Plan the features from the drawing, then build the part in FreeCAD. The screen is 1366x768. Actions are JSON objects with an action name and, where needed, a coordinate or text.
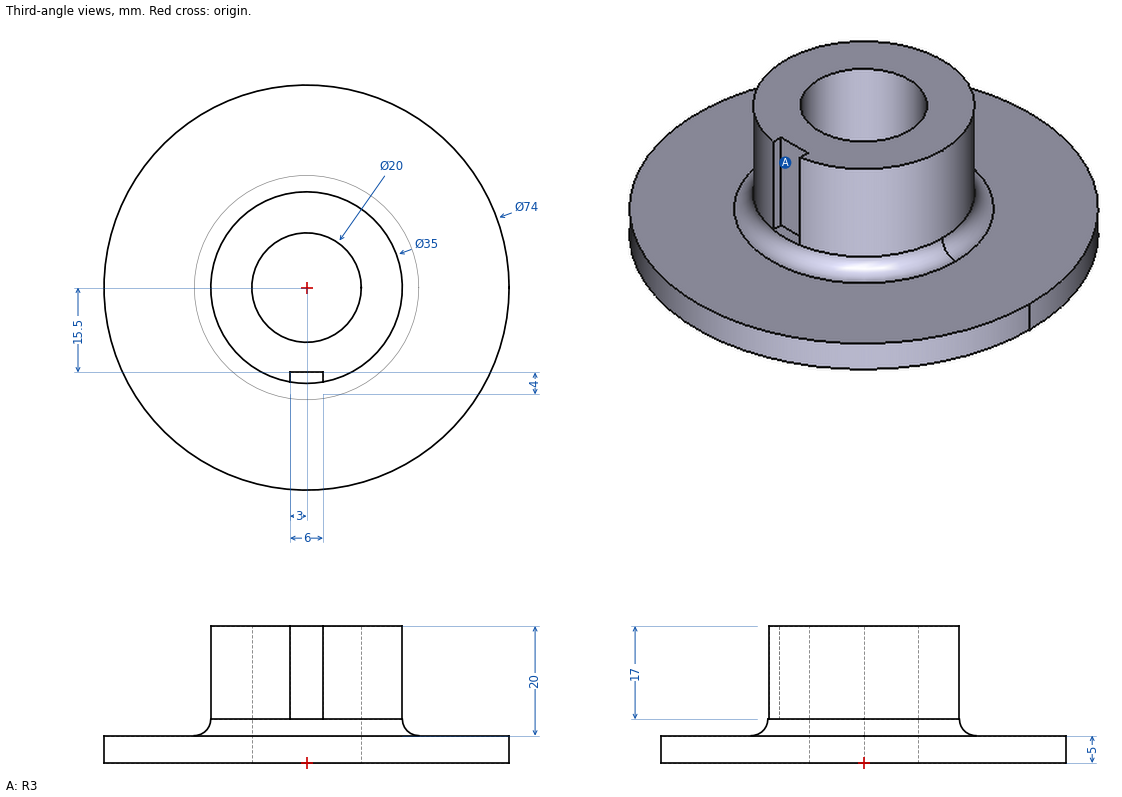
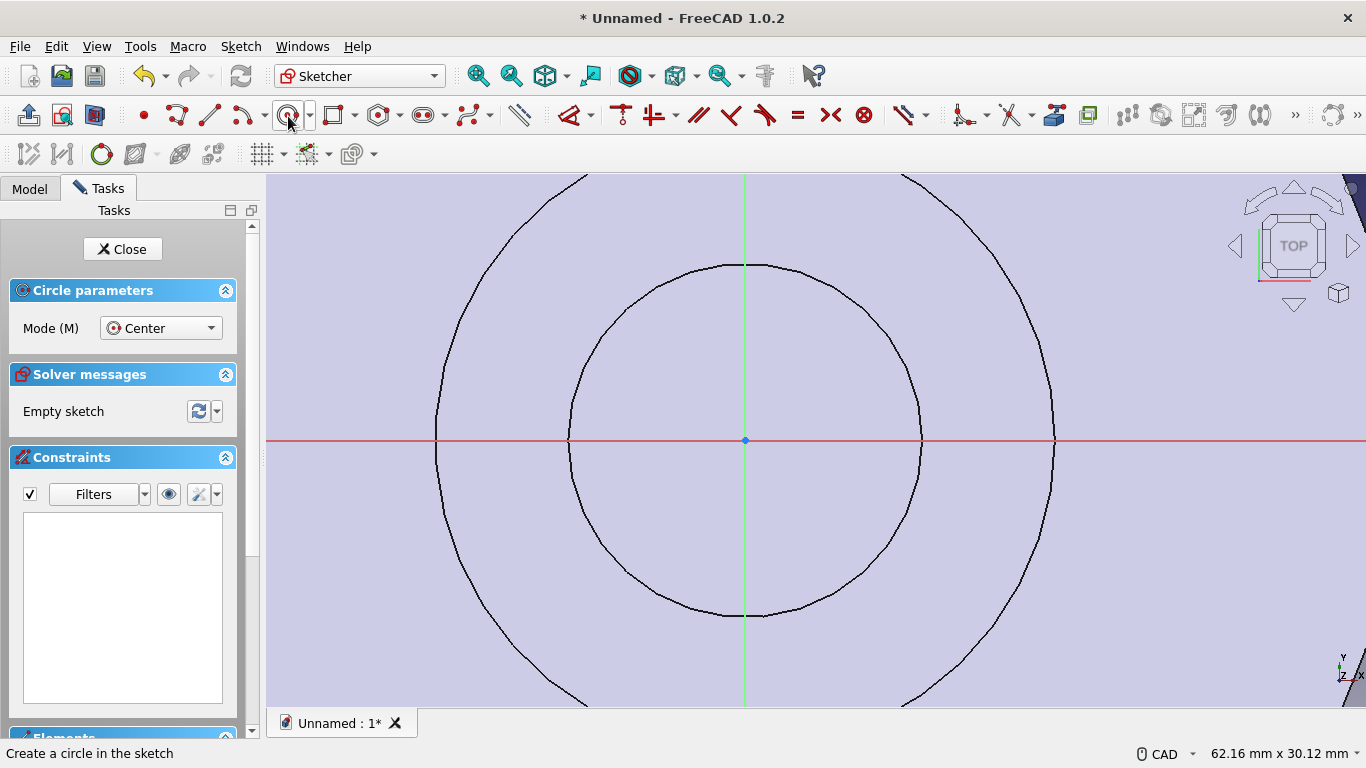
{"action": "left_click", "coordinate": [745, 440]}
{"action": "mouse_move", "coordinate": [870, 315]}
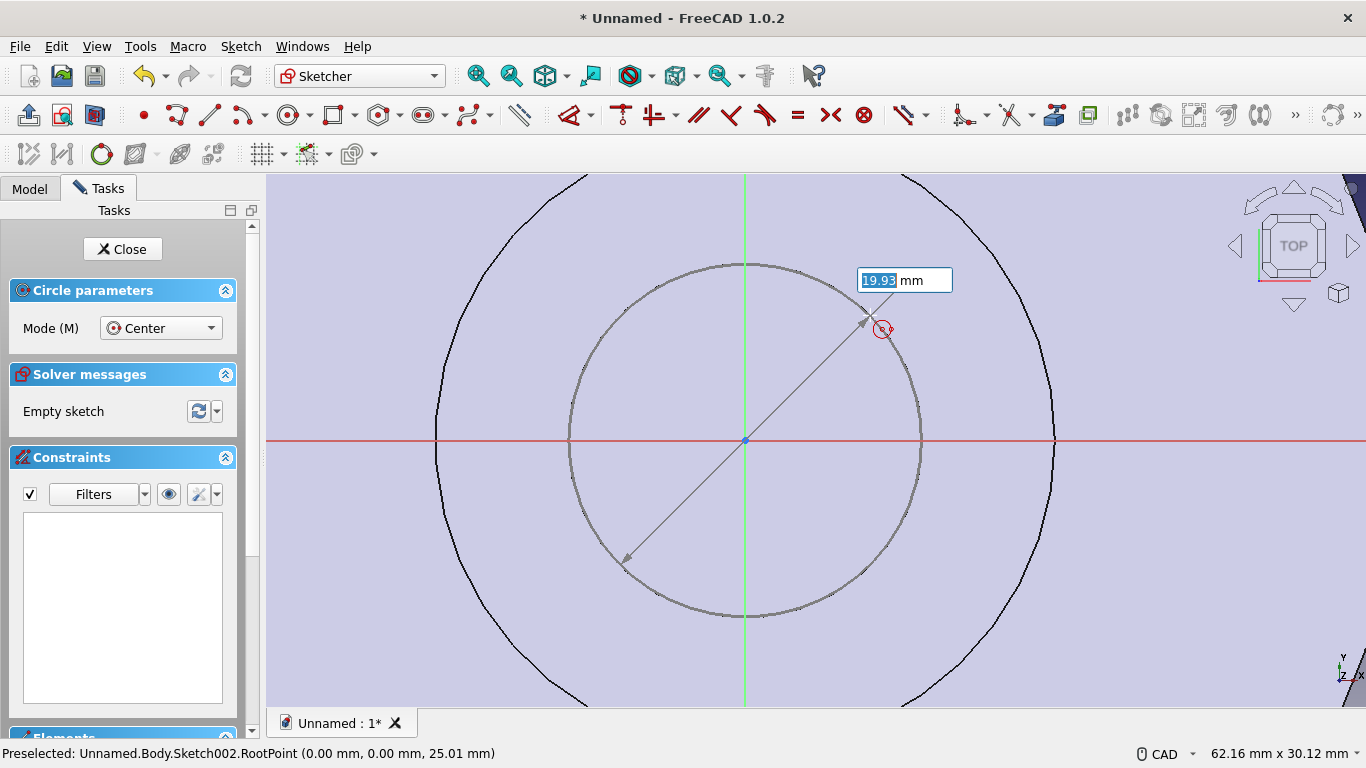
{"action": "type", "text": "20"}
{"action": "key", "text": "Return"}
{"action": "key", "text": "Escape"}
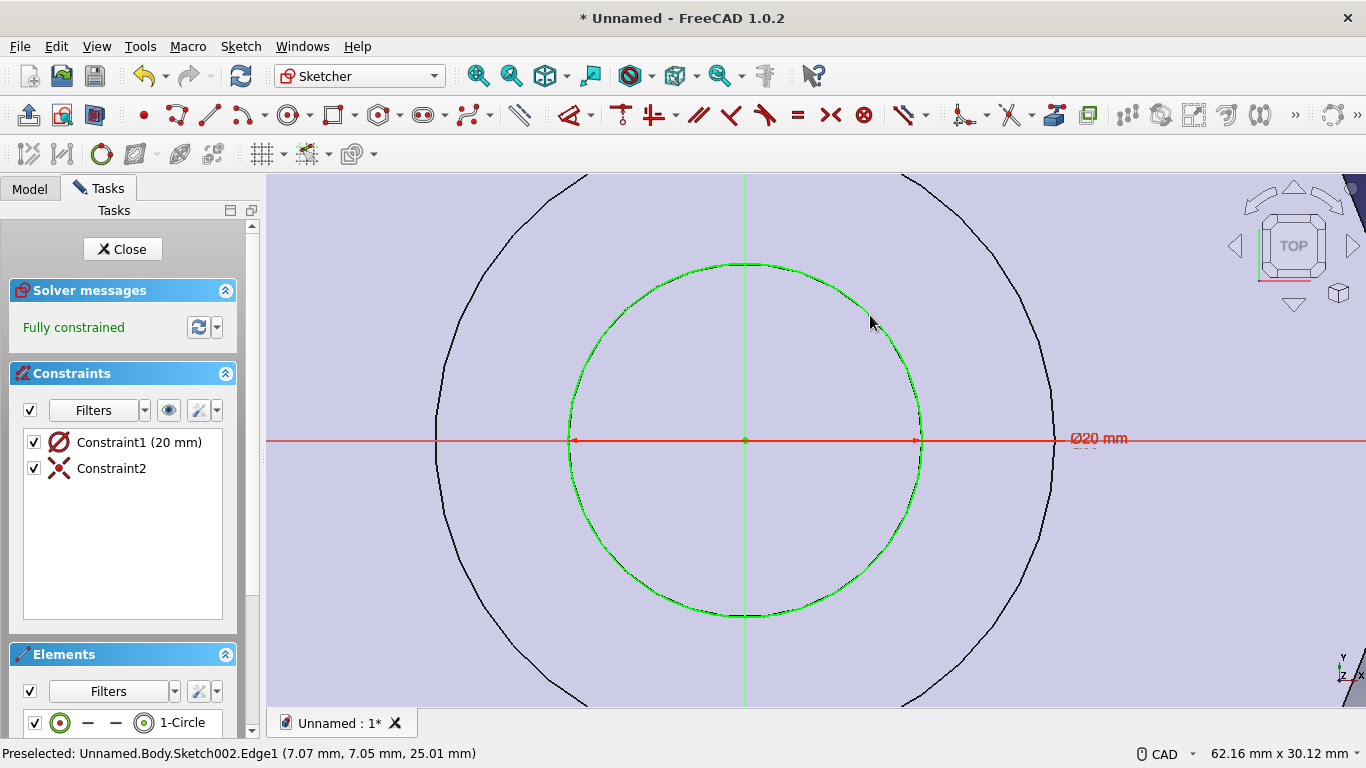
{"action": "left_click", "coordinate": [123, 249]}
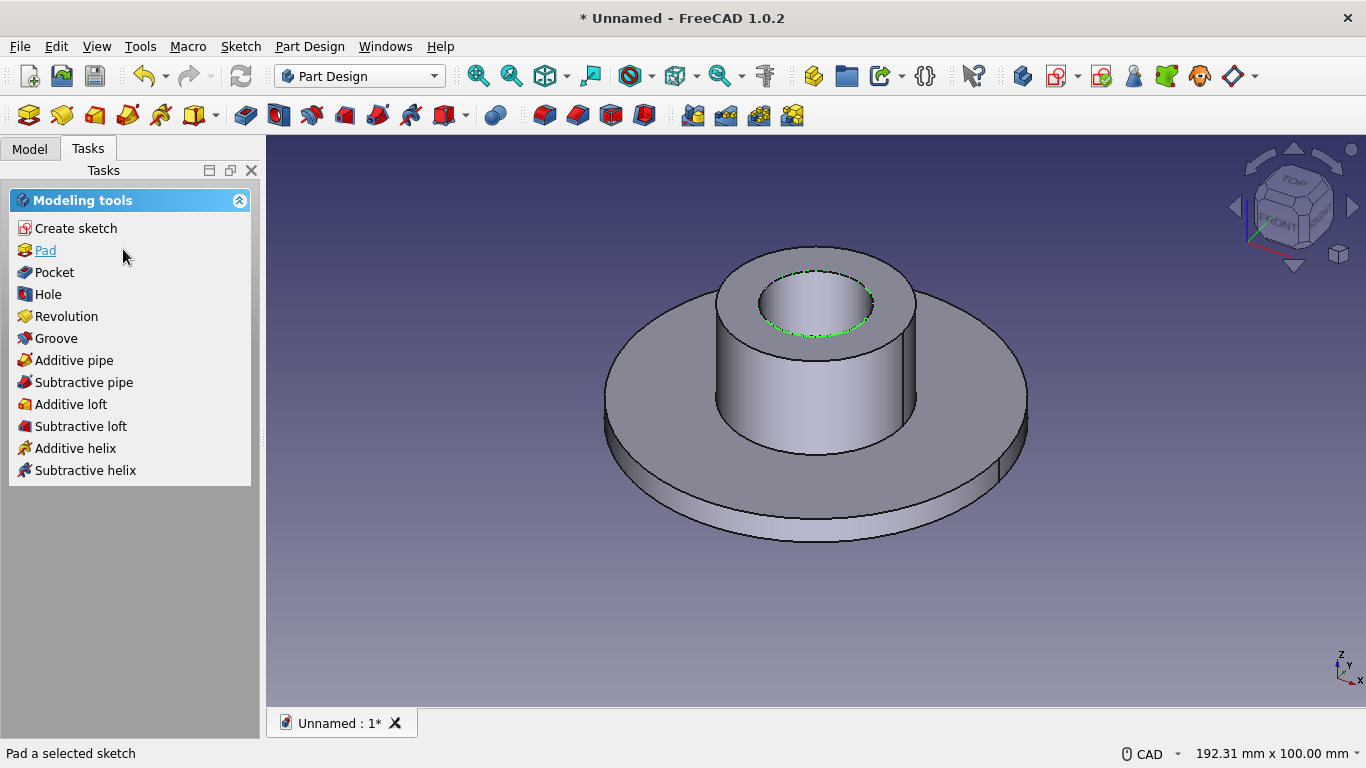
{"action": "left_click", "coordinate": [246, 116]}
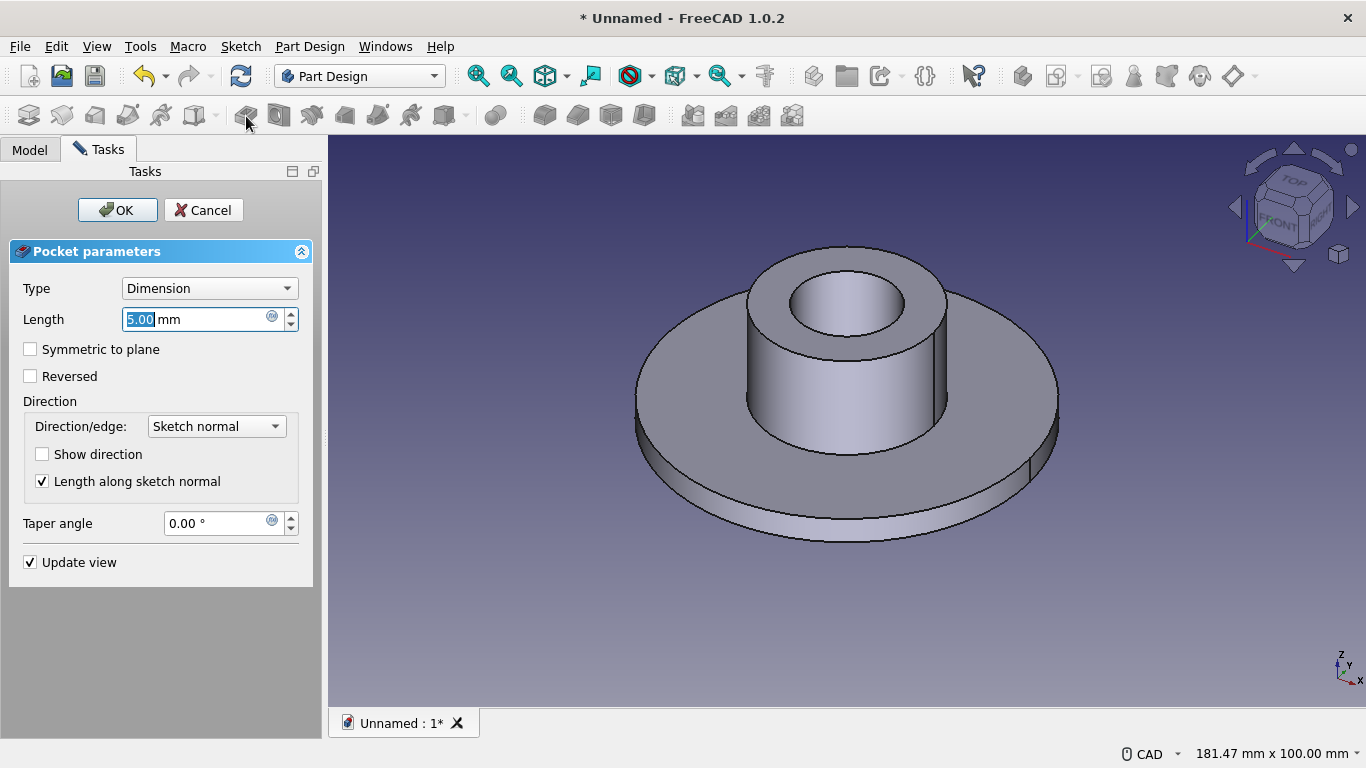
{"action": "left_click", "coordinate": [210, 288]}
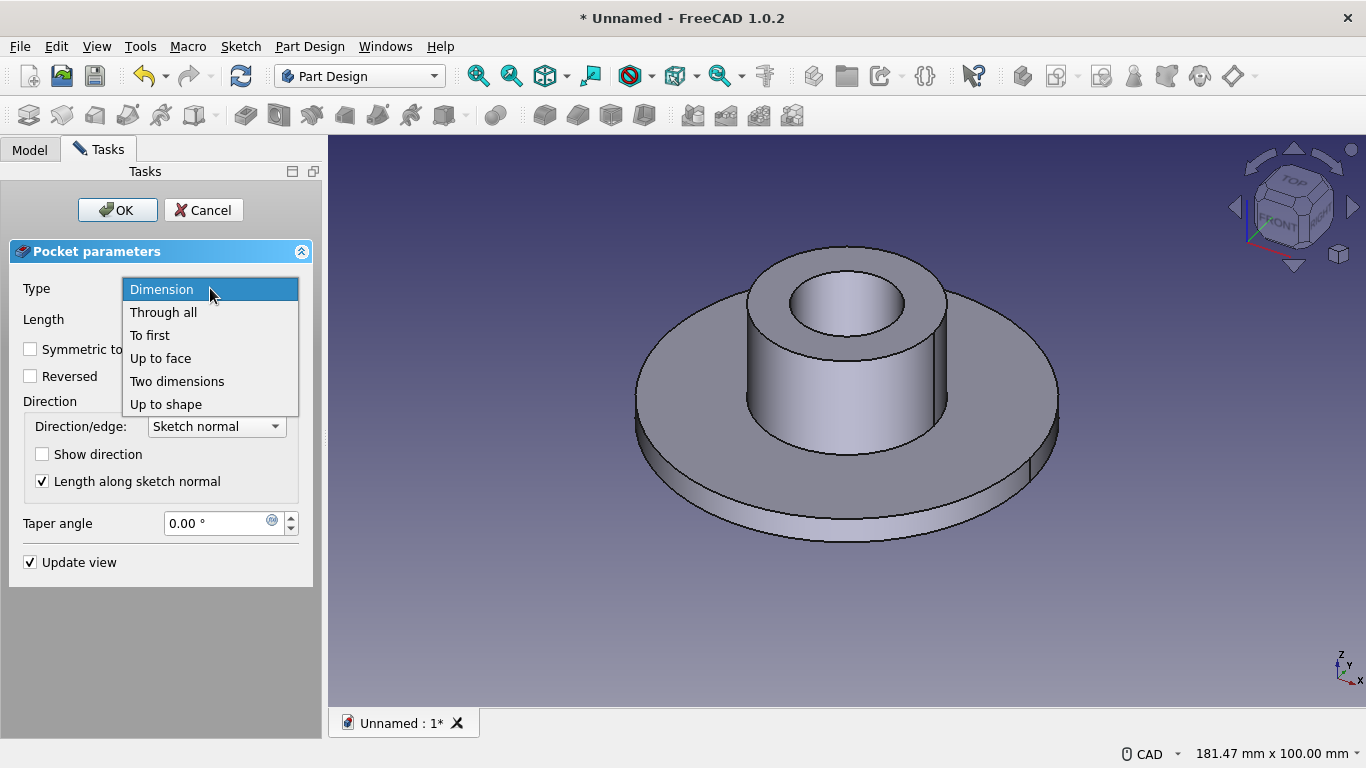
{"action": "left_click", "coordinate": [208, 312]}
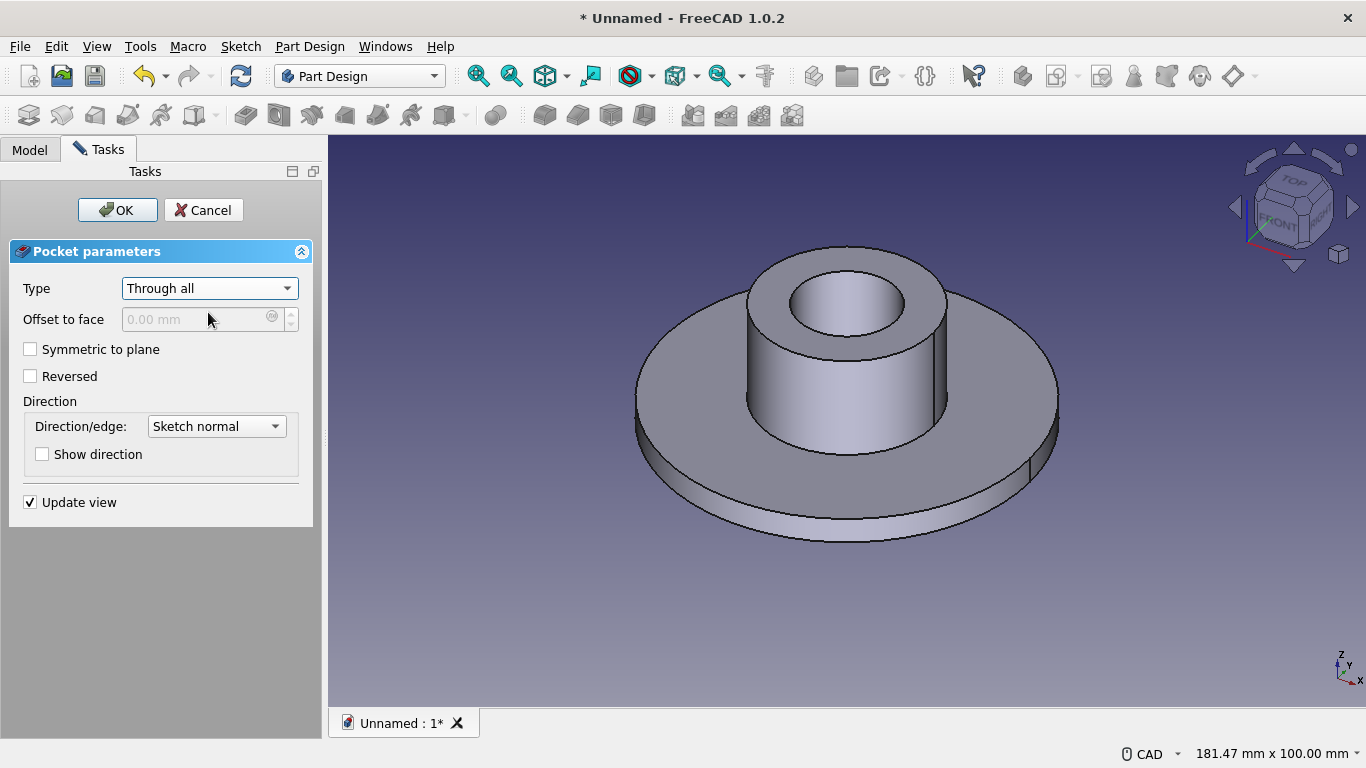
{"action": "left_click", "coordinate": [118, 210]}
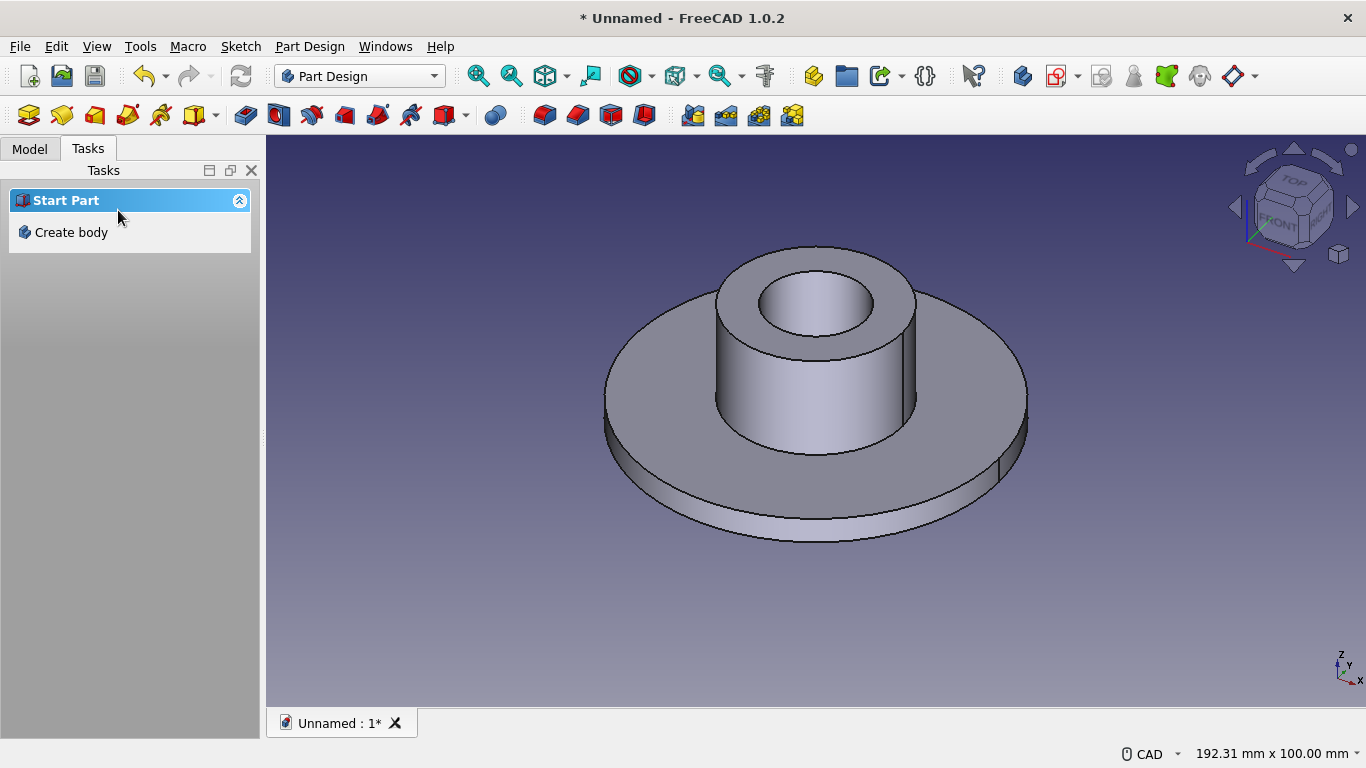
{"action": "key", "text": "0"}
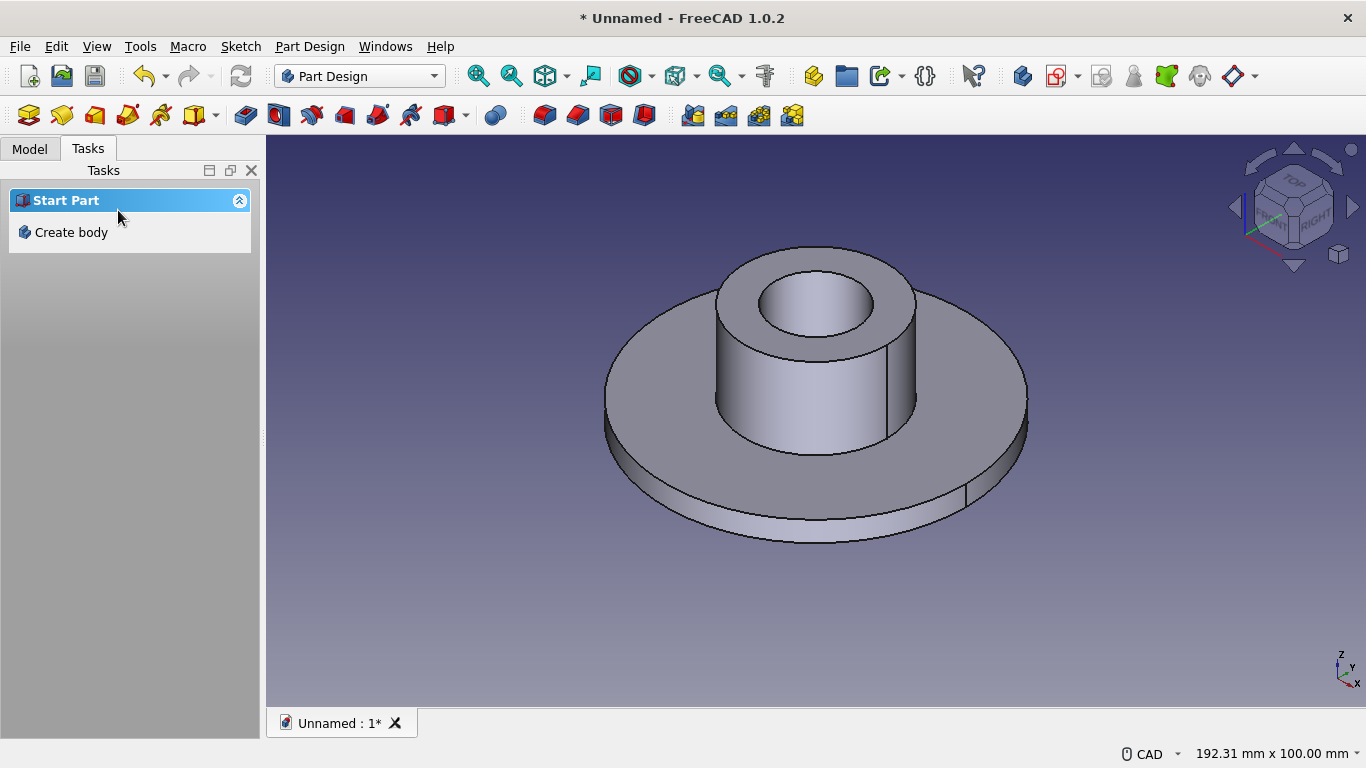
{"action": "left_click", "coordinate": [479, 76]}